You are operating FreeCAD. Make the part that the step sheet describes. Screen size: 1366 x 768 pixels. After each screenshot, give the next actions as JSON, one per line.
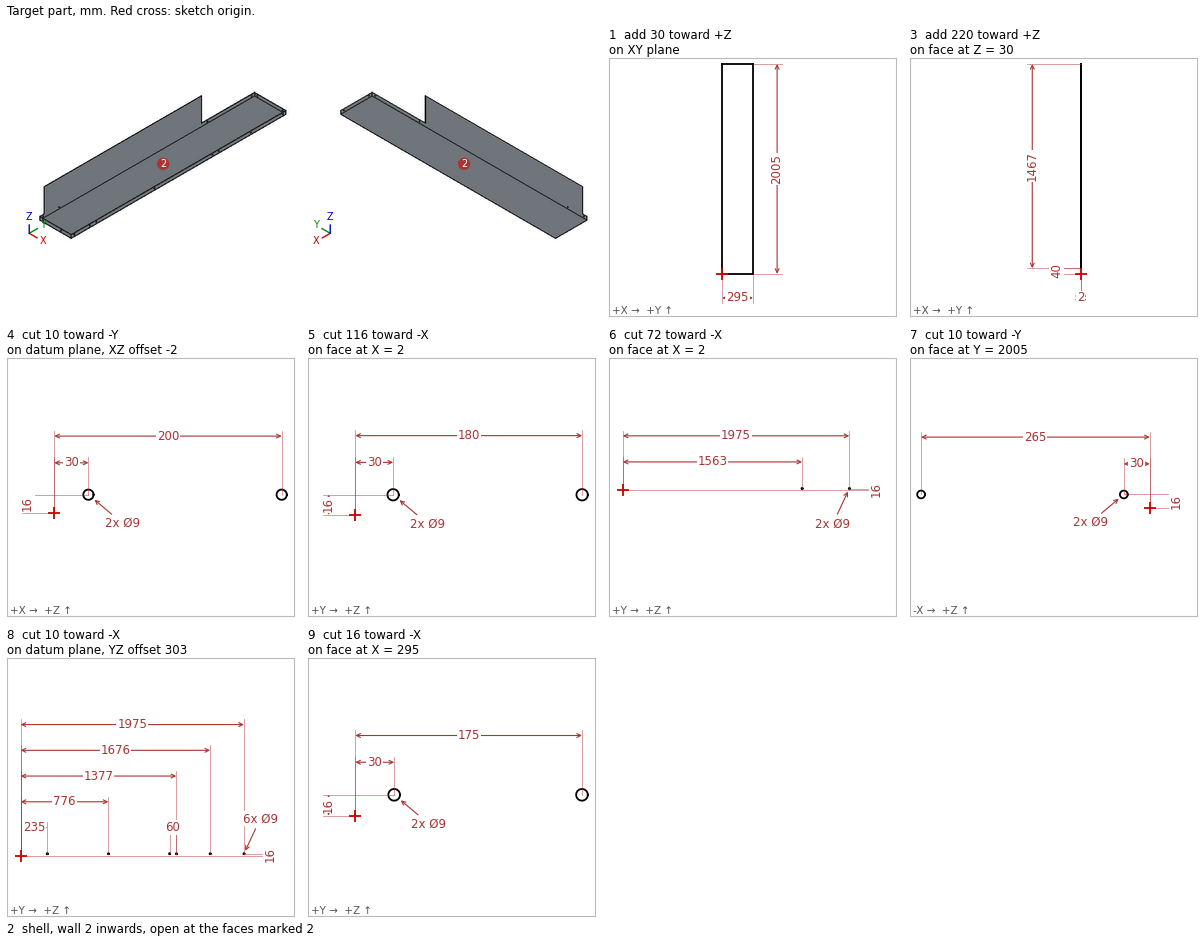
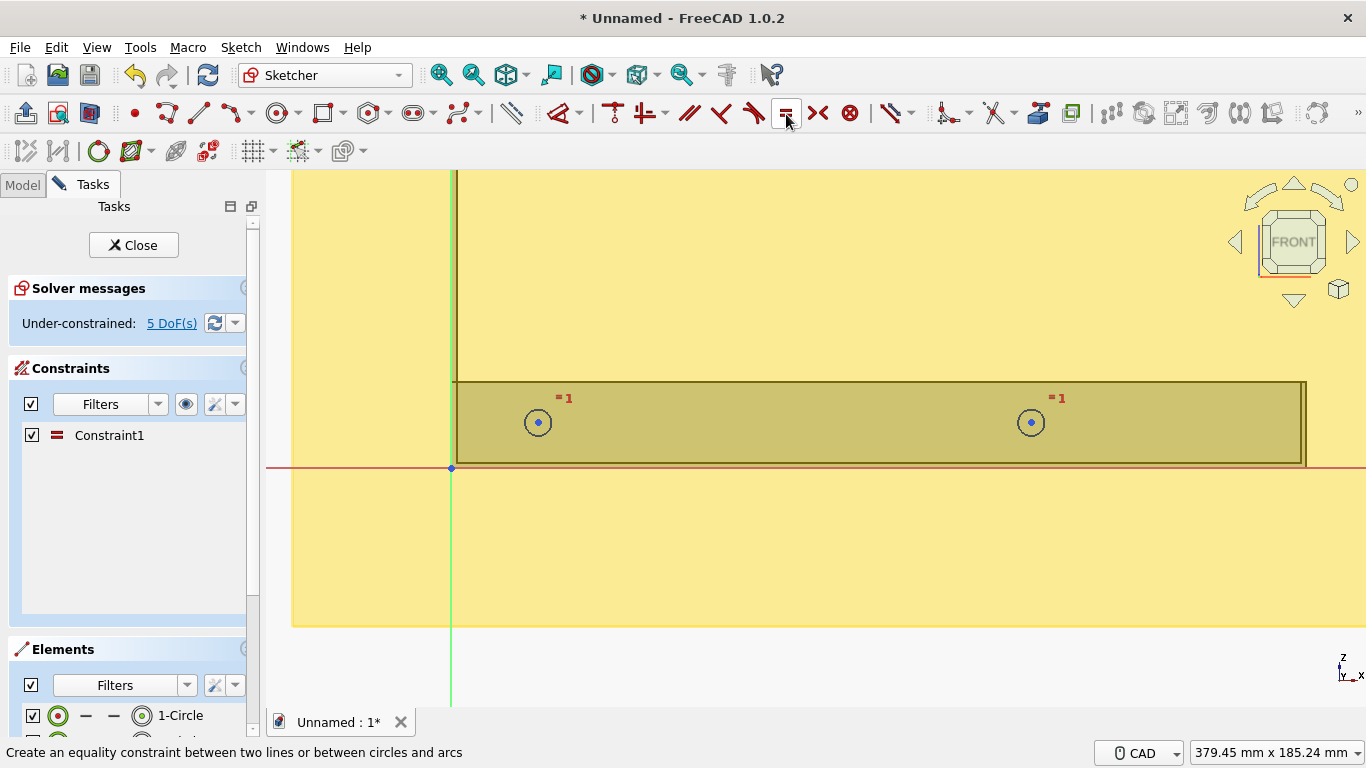
{"action": "left_click", "coordinate": [538, 423]}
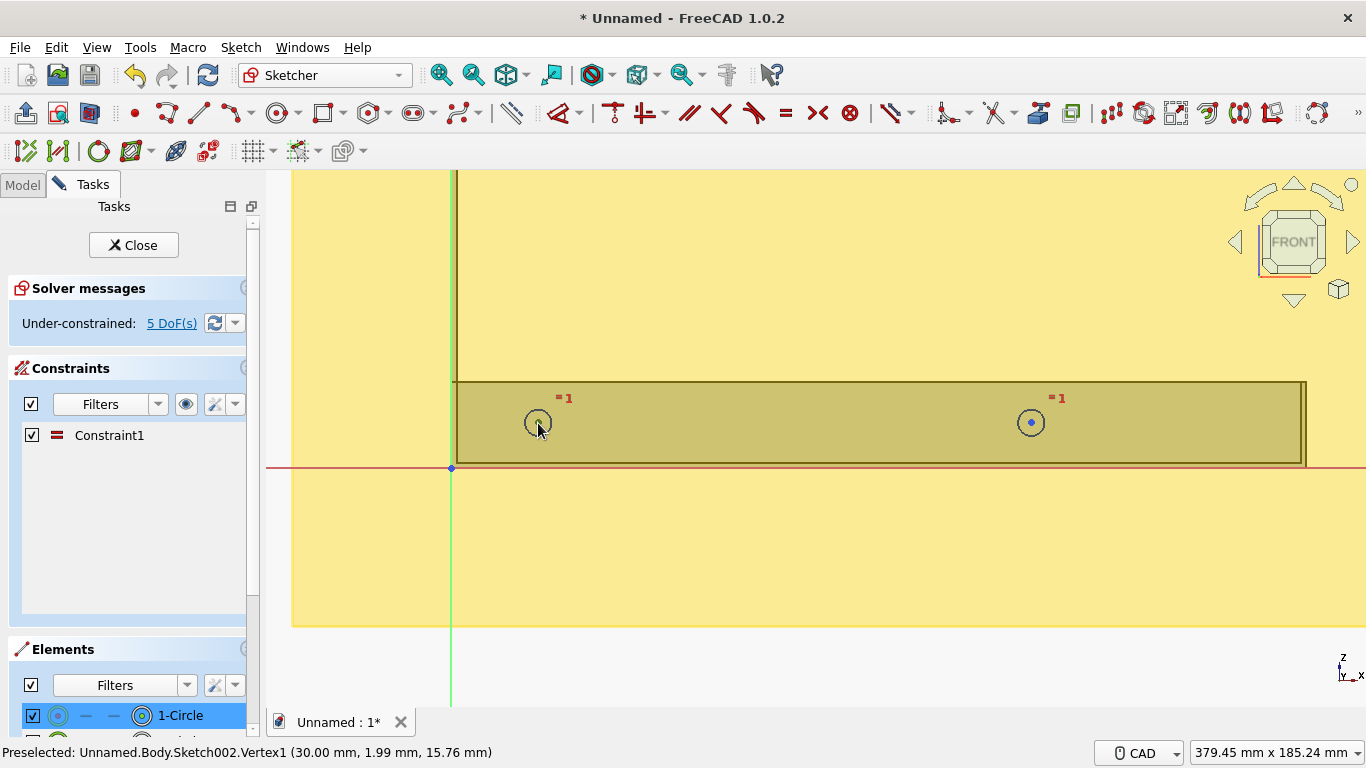
{"action": "left_click", "coordinate": [1031, 423]}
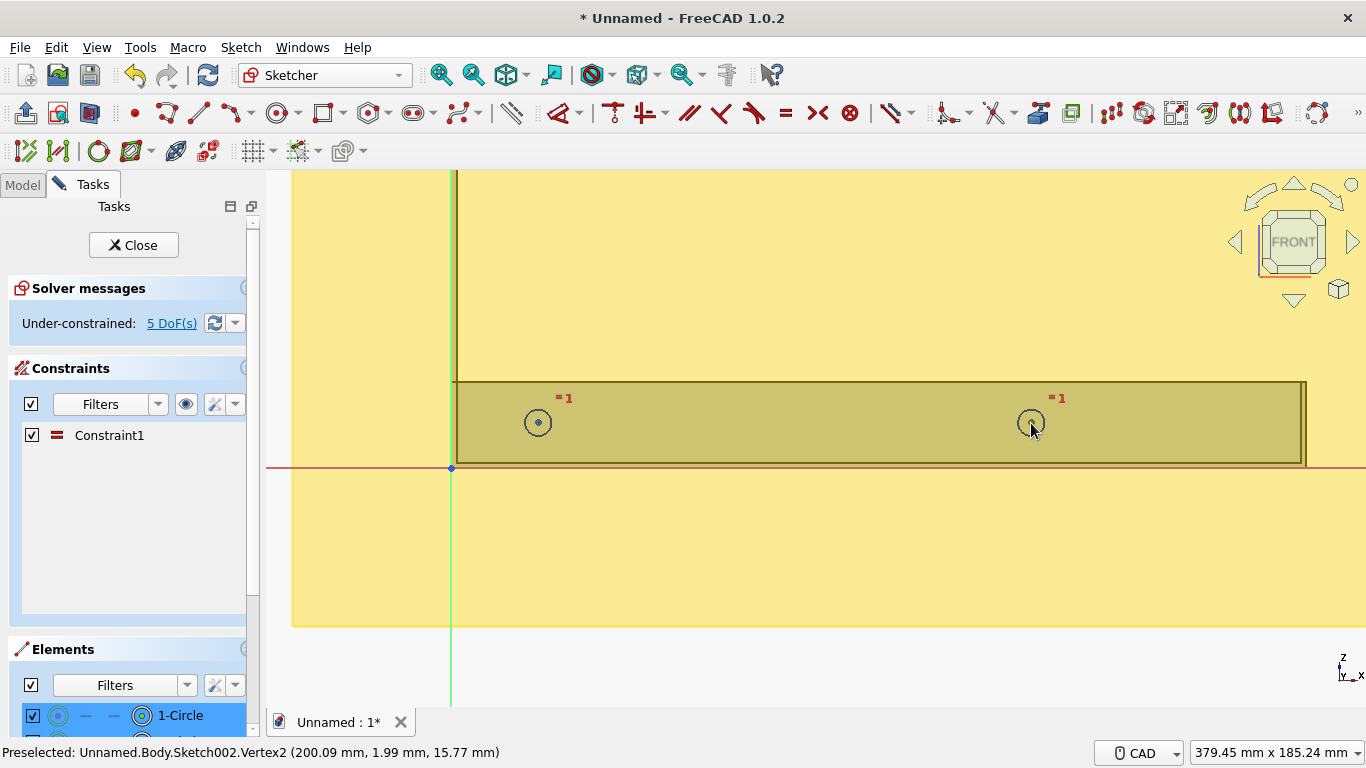
{"action": "left_click", "coordinate": [668, 114]}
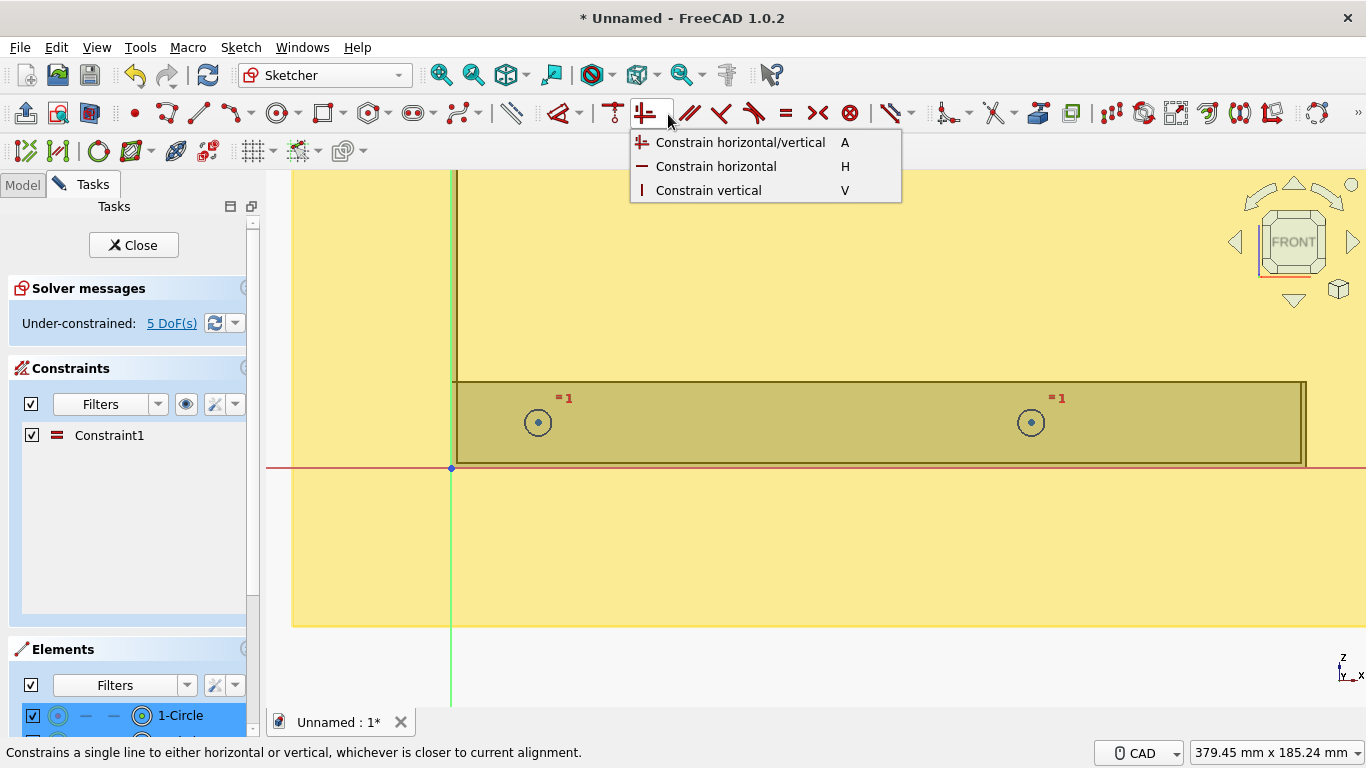
{"action": "left_click", "coordinate": [766, 166]}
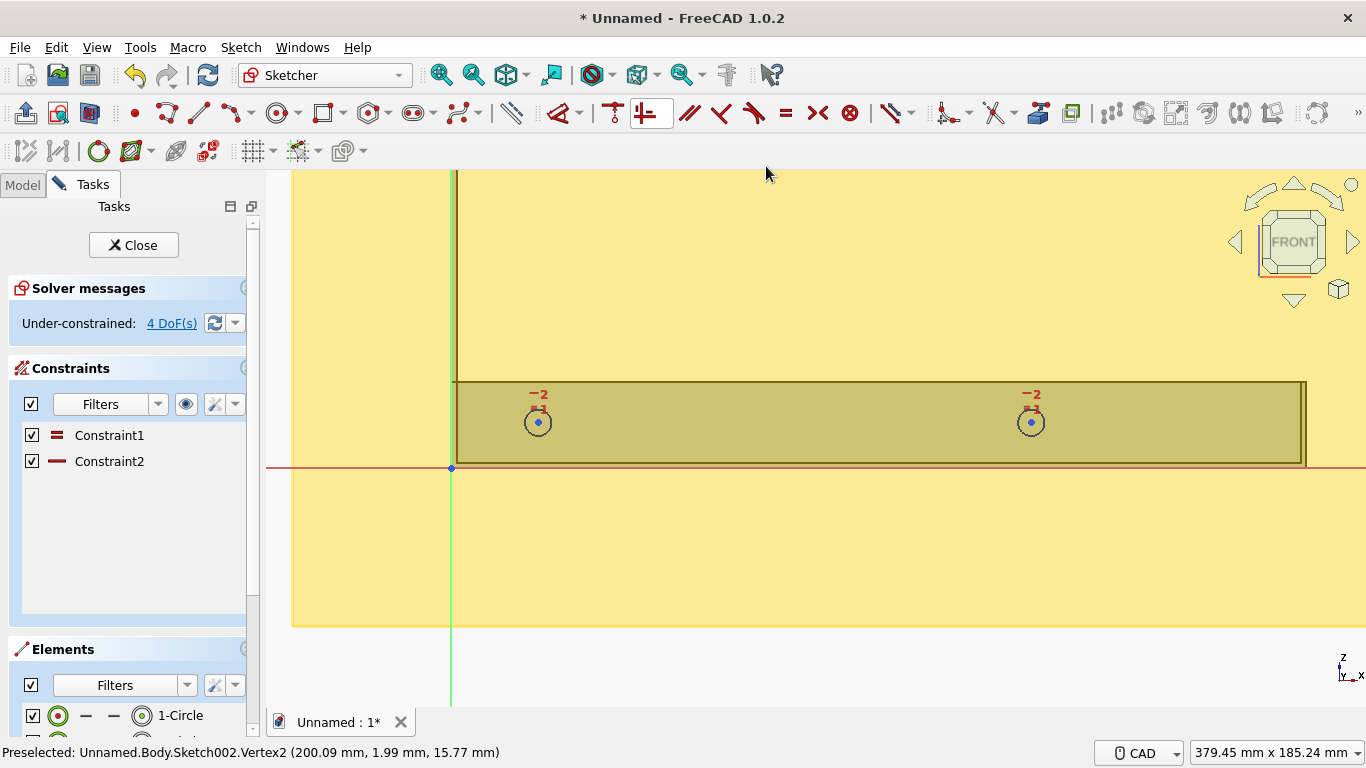
{"action": "left_click", "coordinate": [558, 114]}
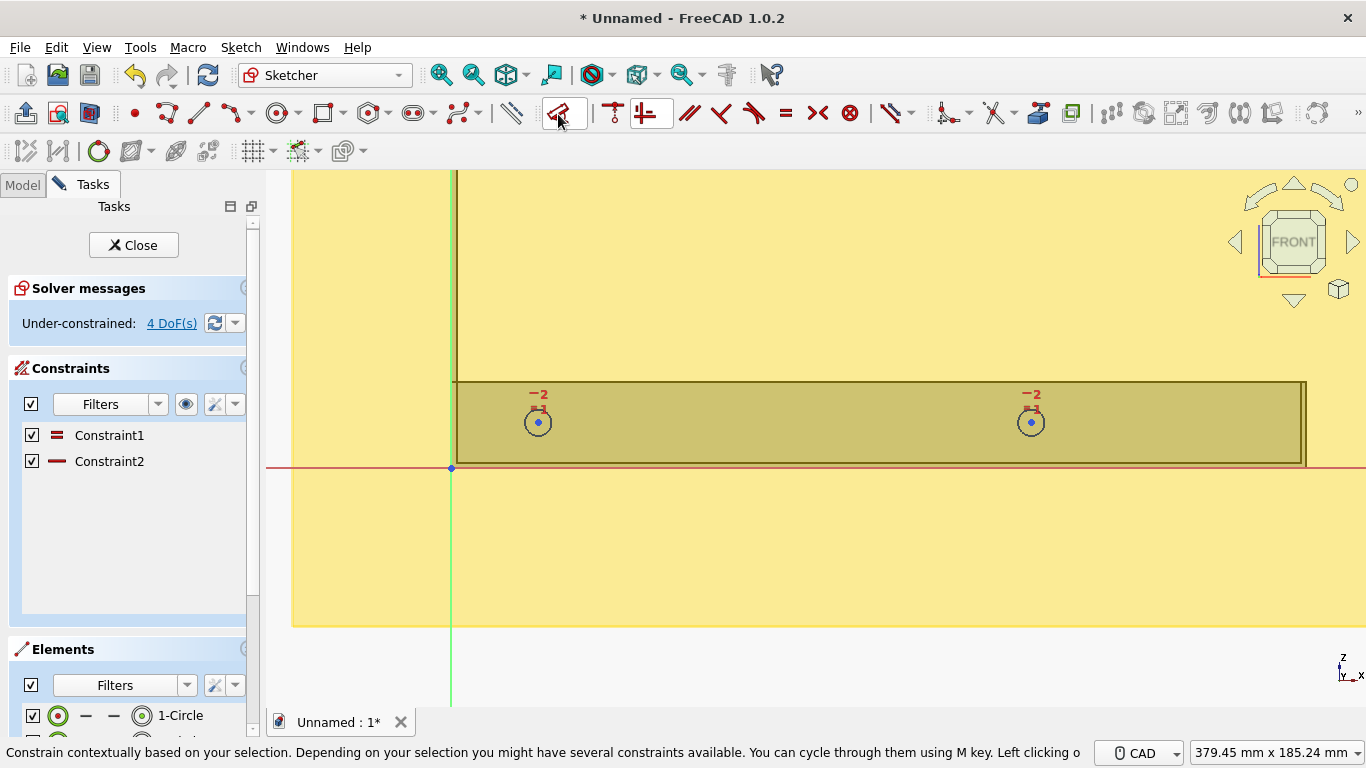
{"action": "scroll", "coordinate": [548, 413], "scroll_direction": "up", "scroll_amount": 3}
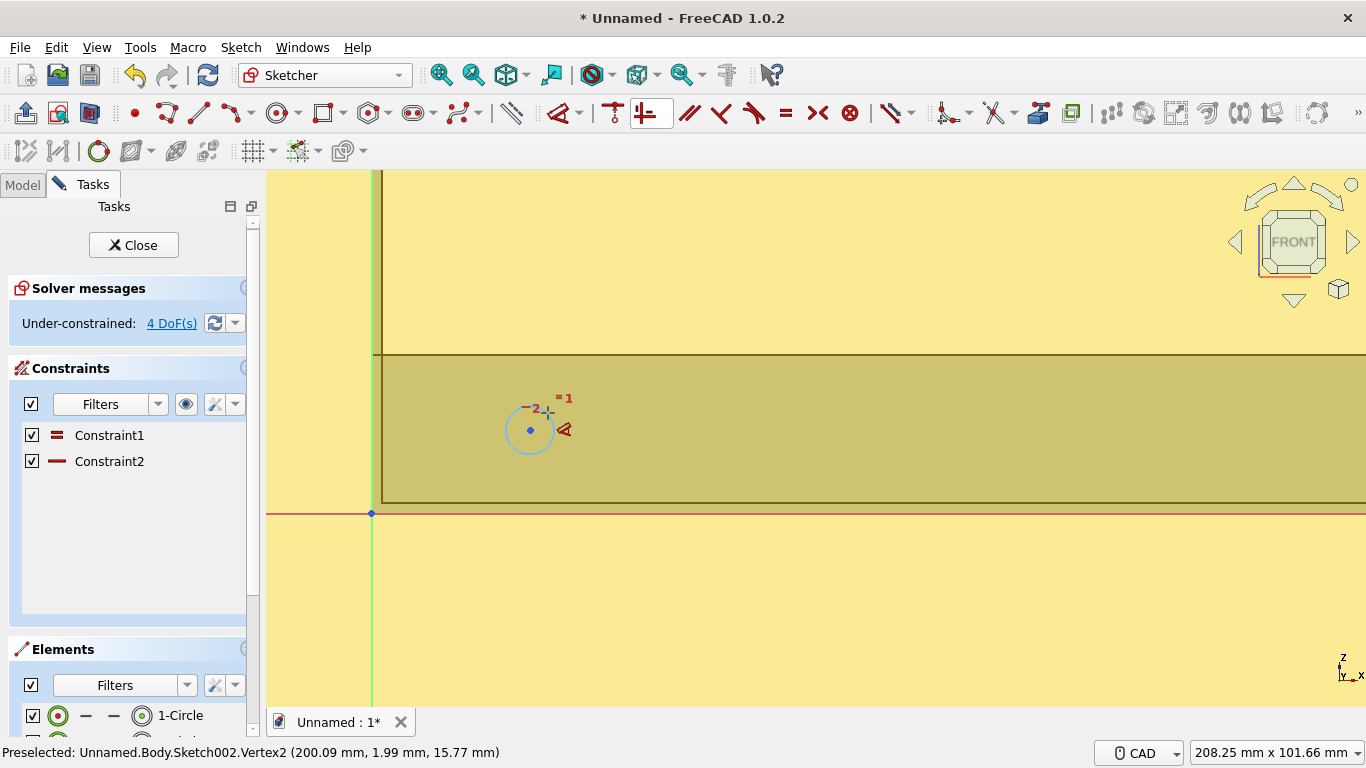
{"action": "left_click", "coordinate": [547, 413]}
{"action": "left_click", "coordinate": [569, 390]}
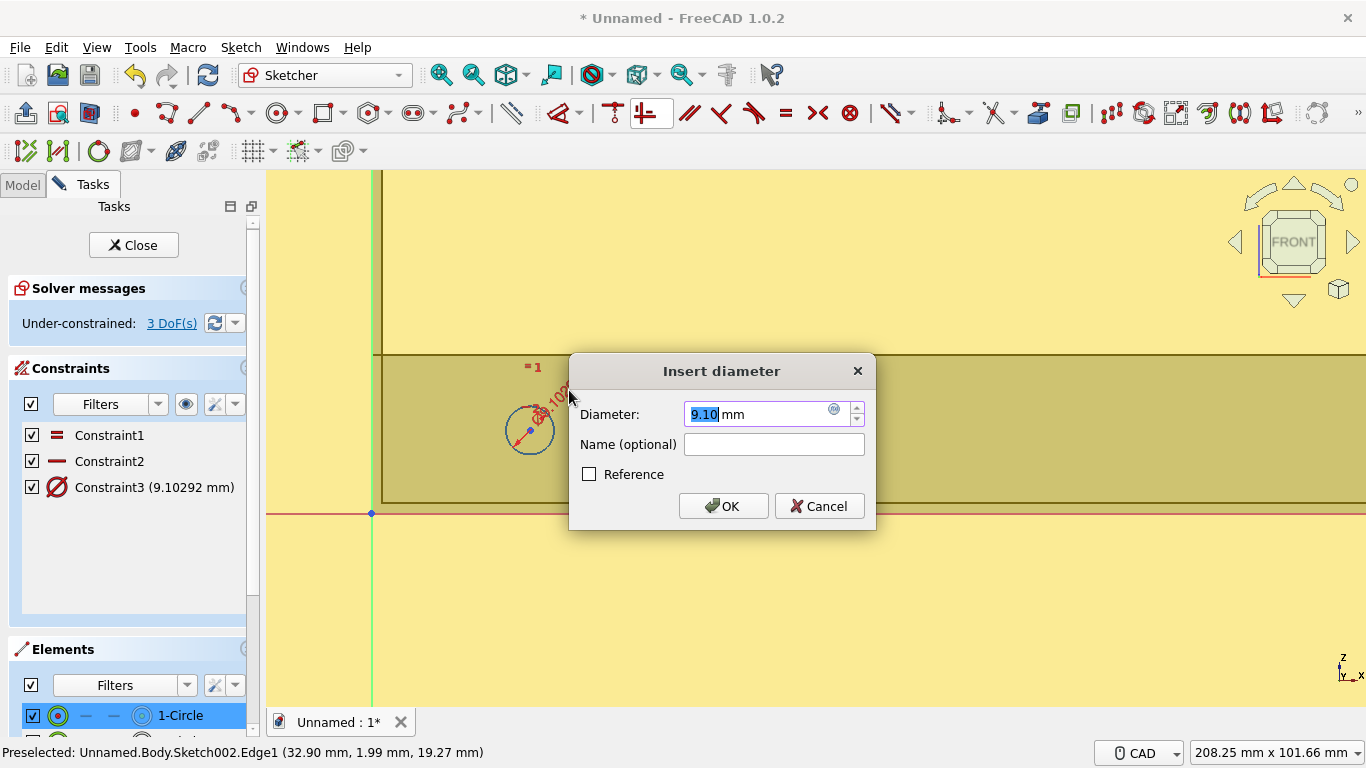
{"action": "type", "text": "9"}
{"action": "key", "text": "Return"}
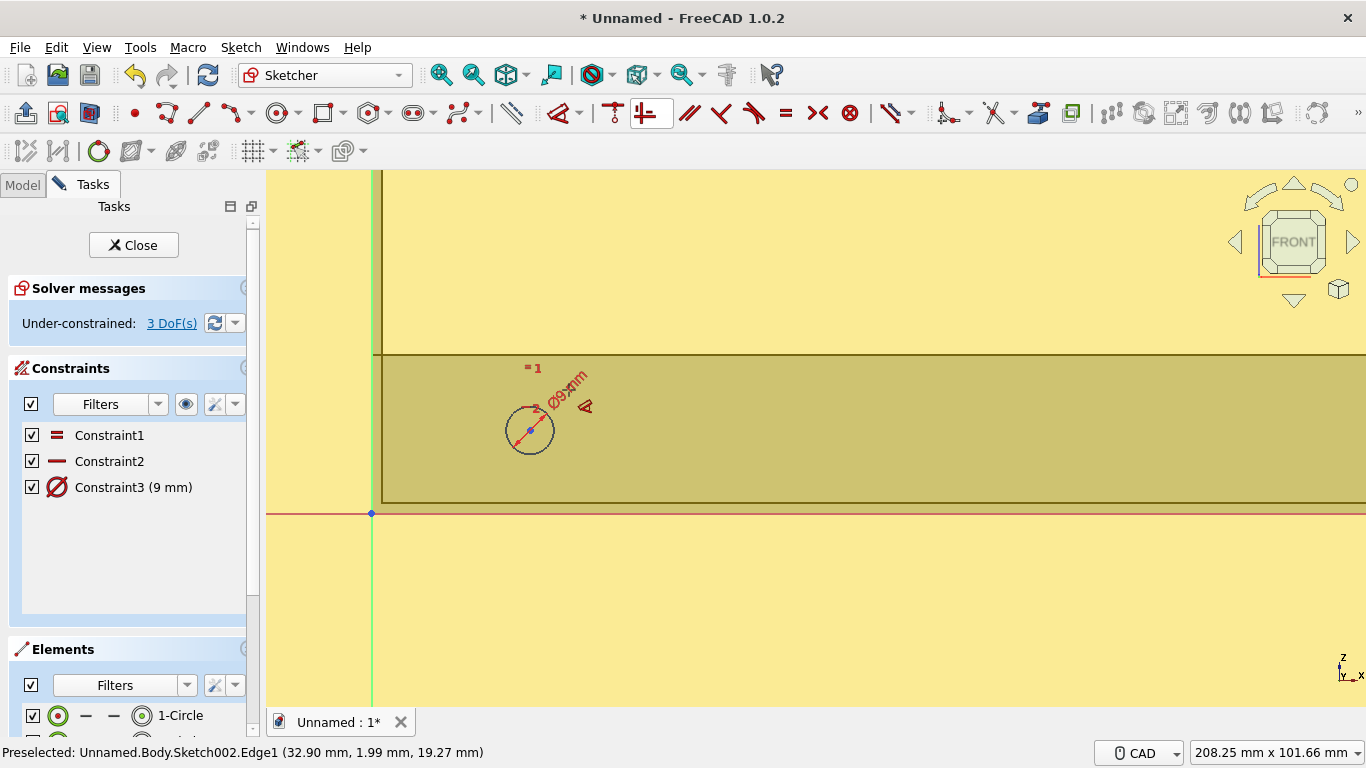
{"action": "left_click", "coordinate": [530, 430]}
{"action": "left_click", "coordinate": [451, 548]}